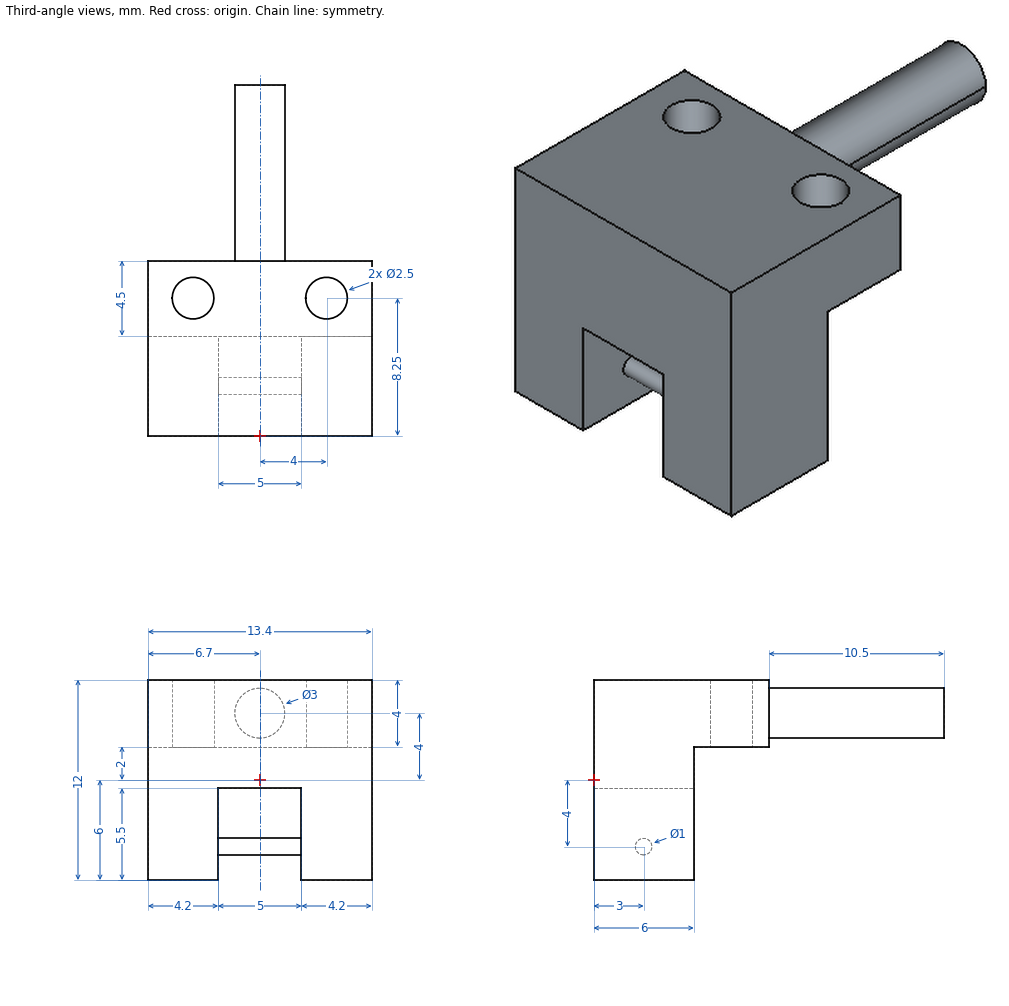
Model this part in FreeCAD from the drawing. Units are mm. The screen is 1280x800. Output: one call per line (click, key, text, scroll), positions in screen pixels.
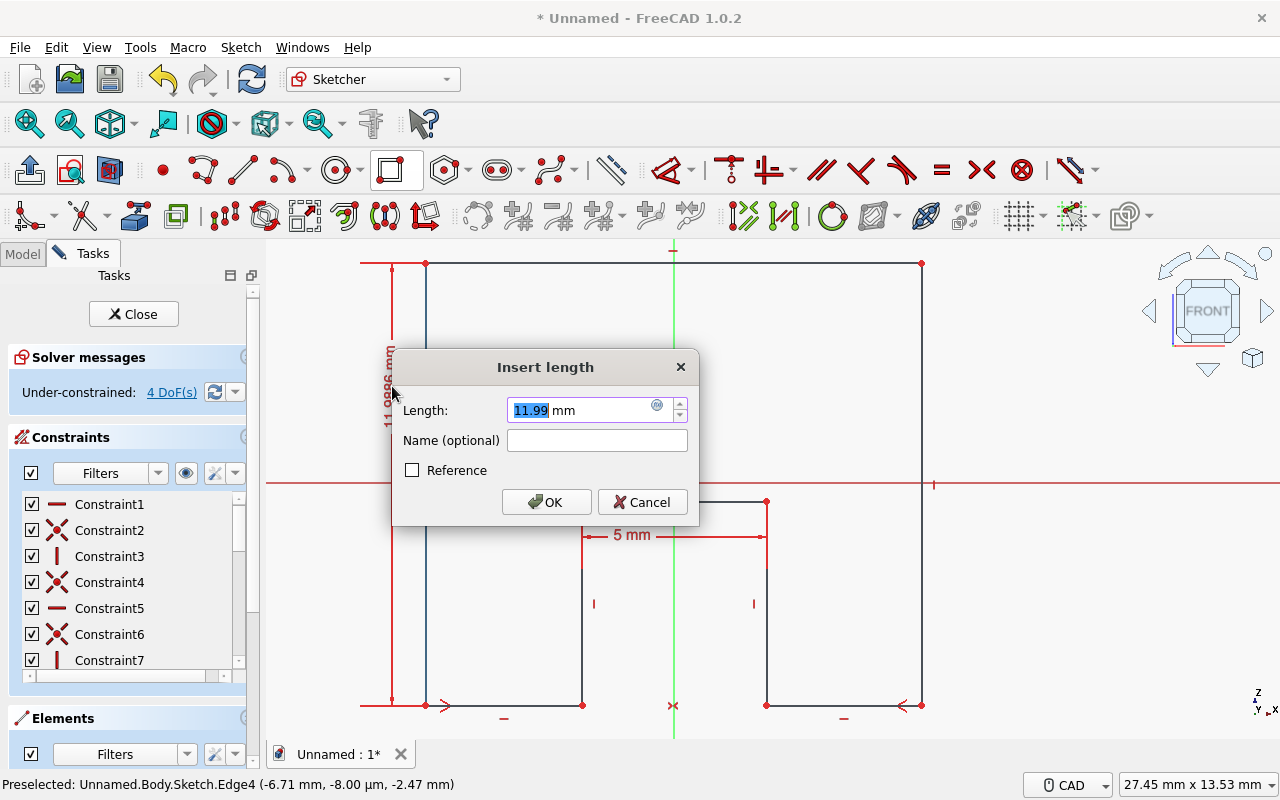
text(12)
key(Return)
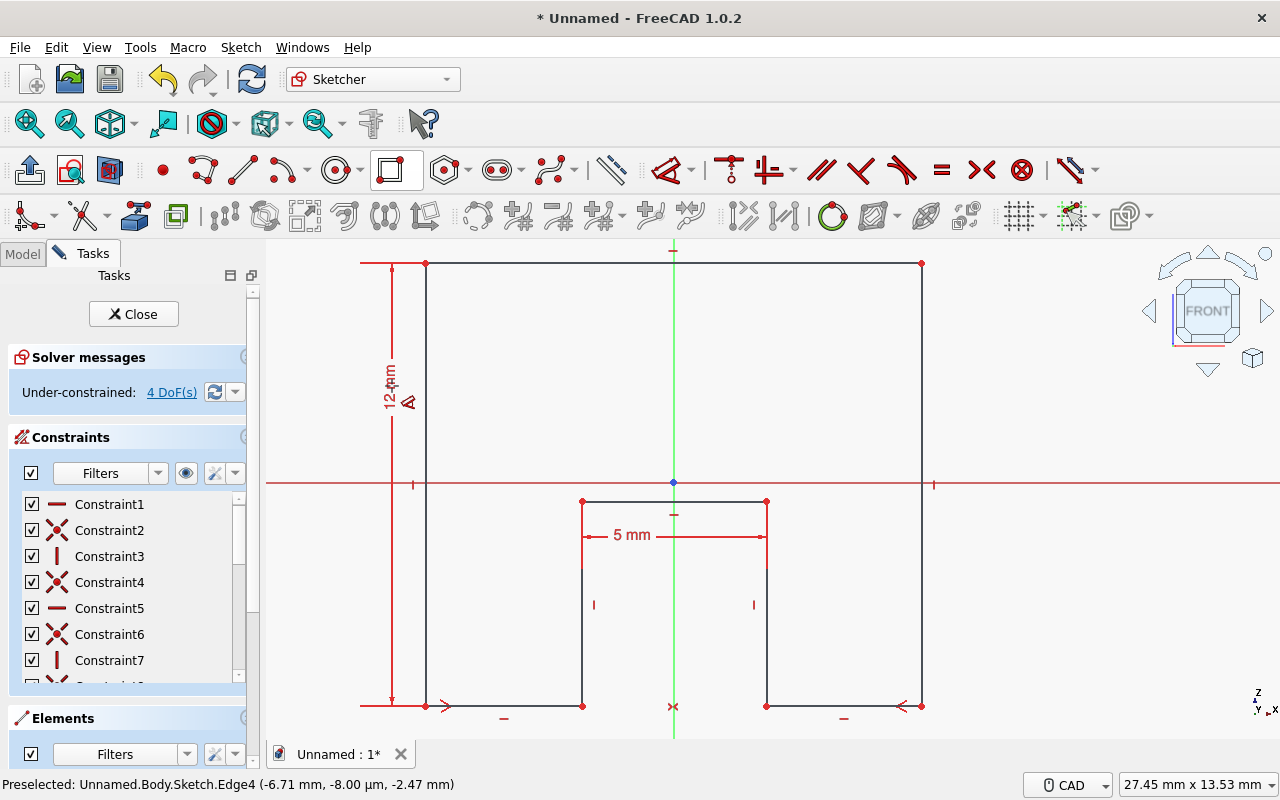
click(582, 706)
click(548, 595)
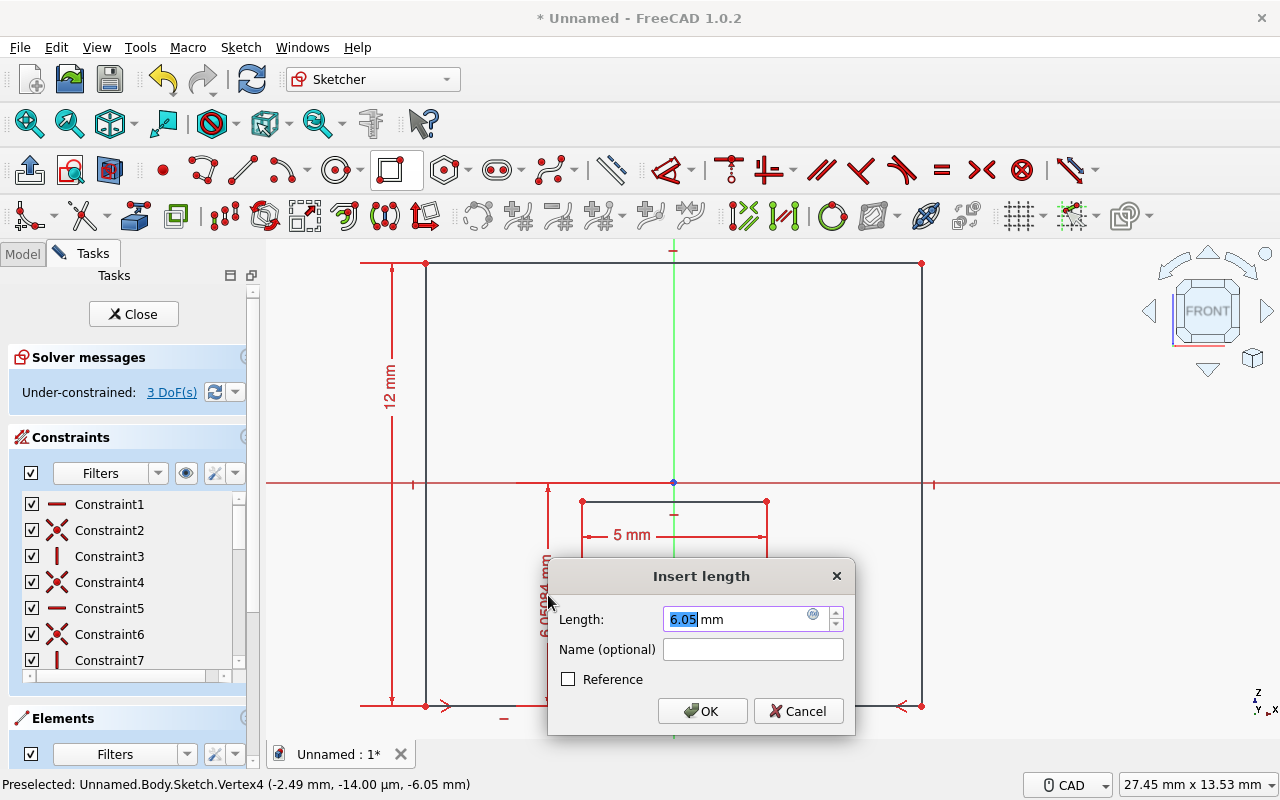
text(6)
key(Return)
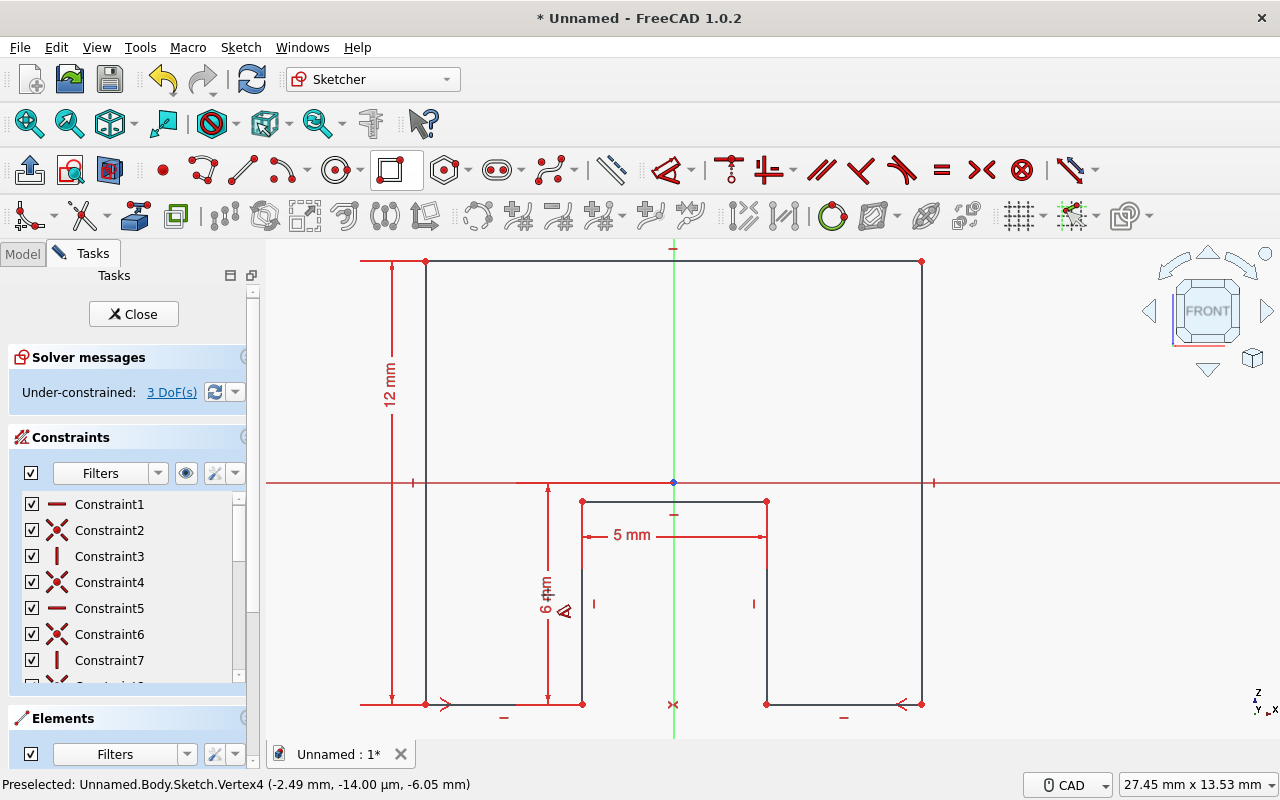
click(582, 563)
click(548, 557)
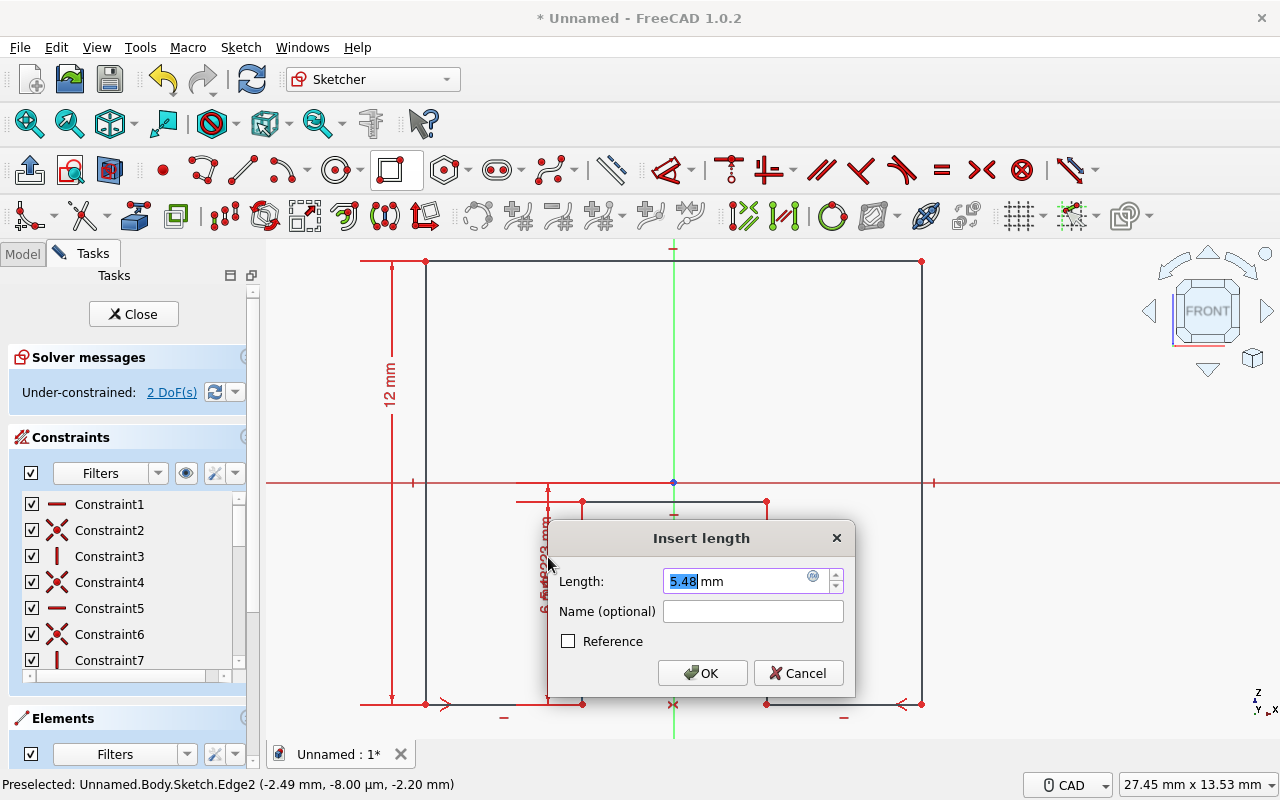
text(5.5)
key(Return)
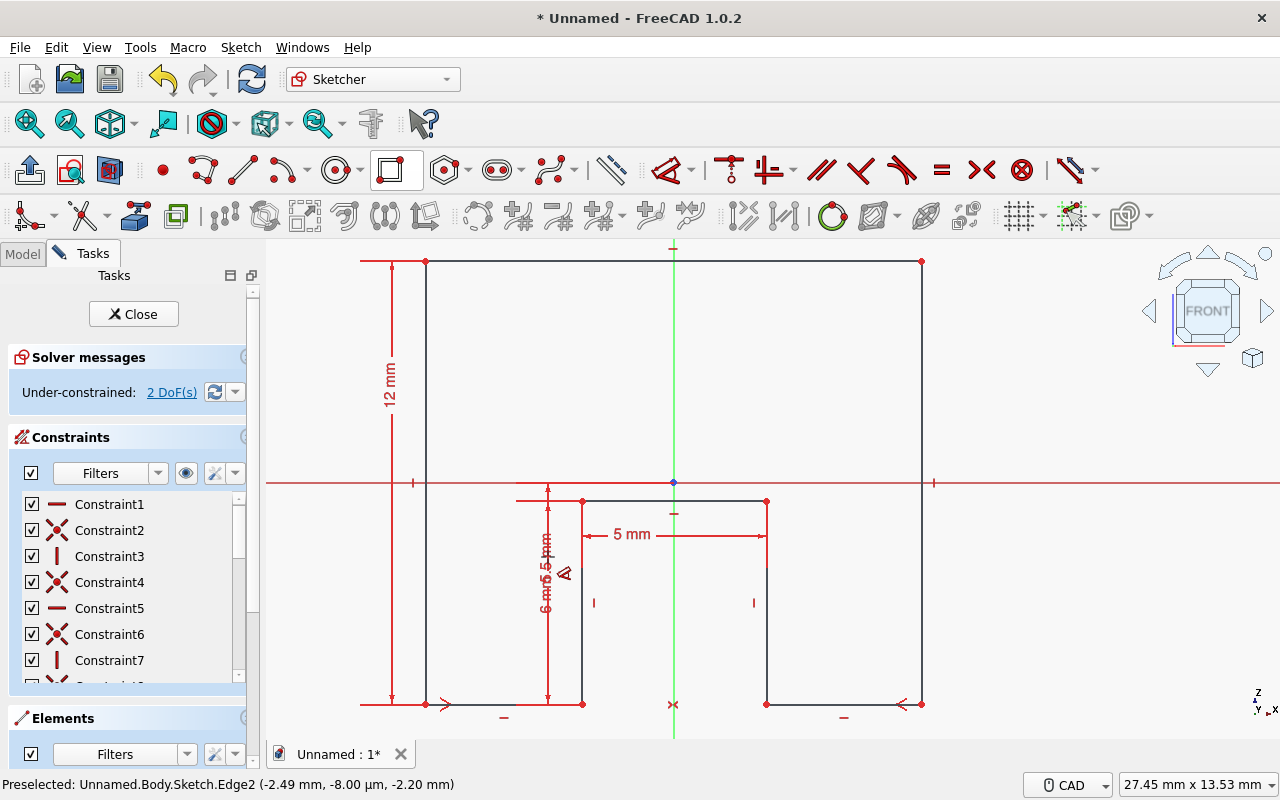
click(535, 705)
click(504, 671)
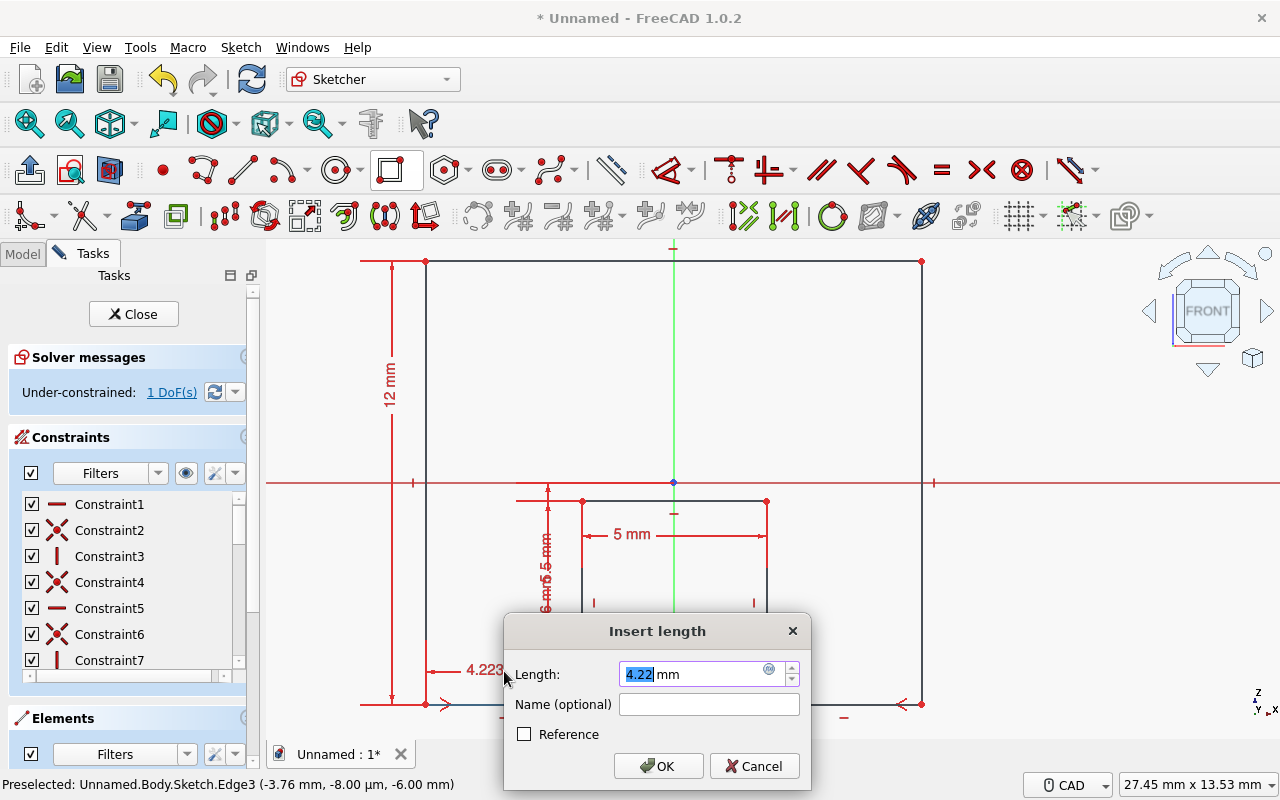
text(4.2)
key(Return)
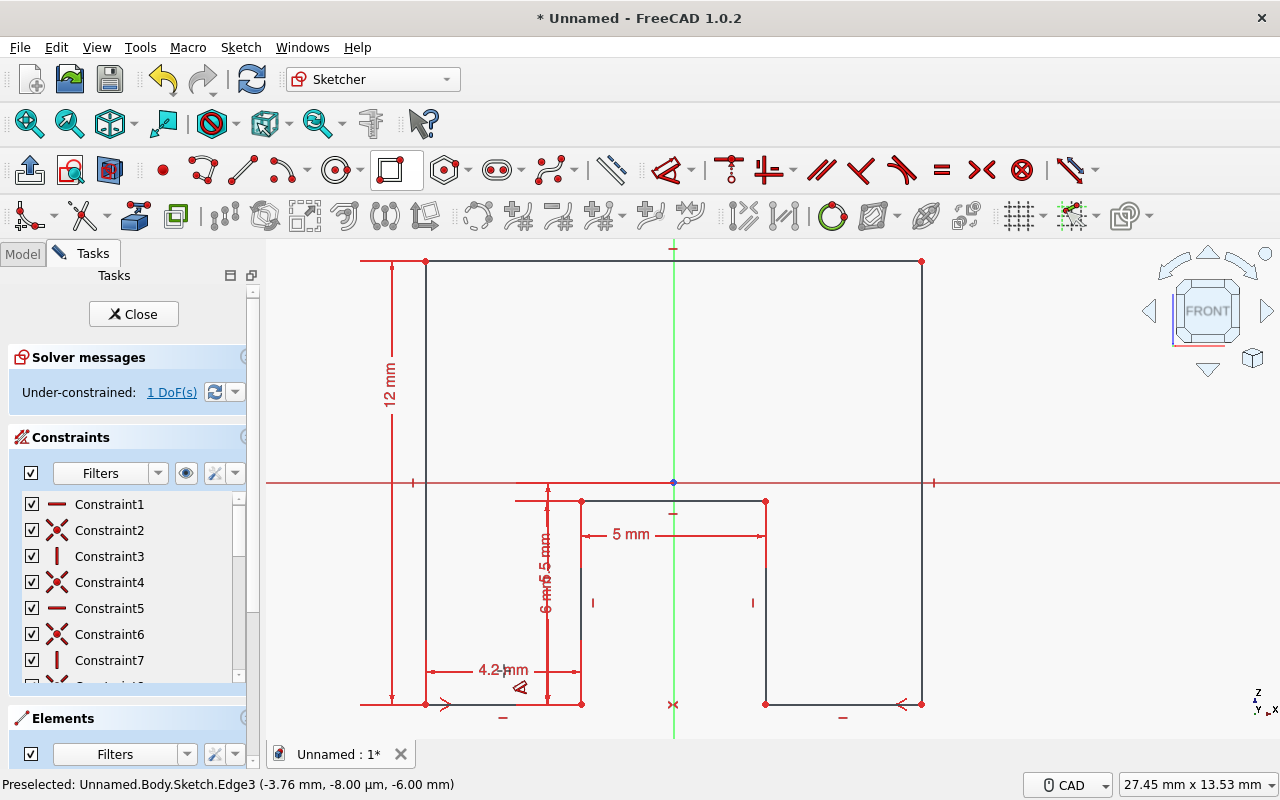
click(875, 705)
click(844, 671)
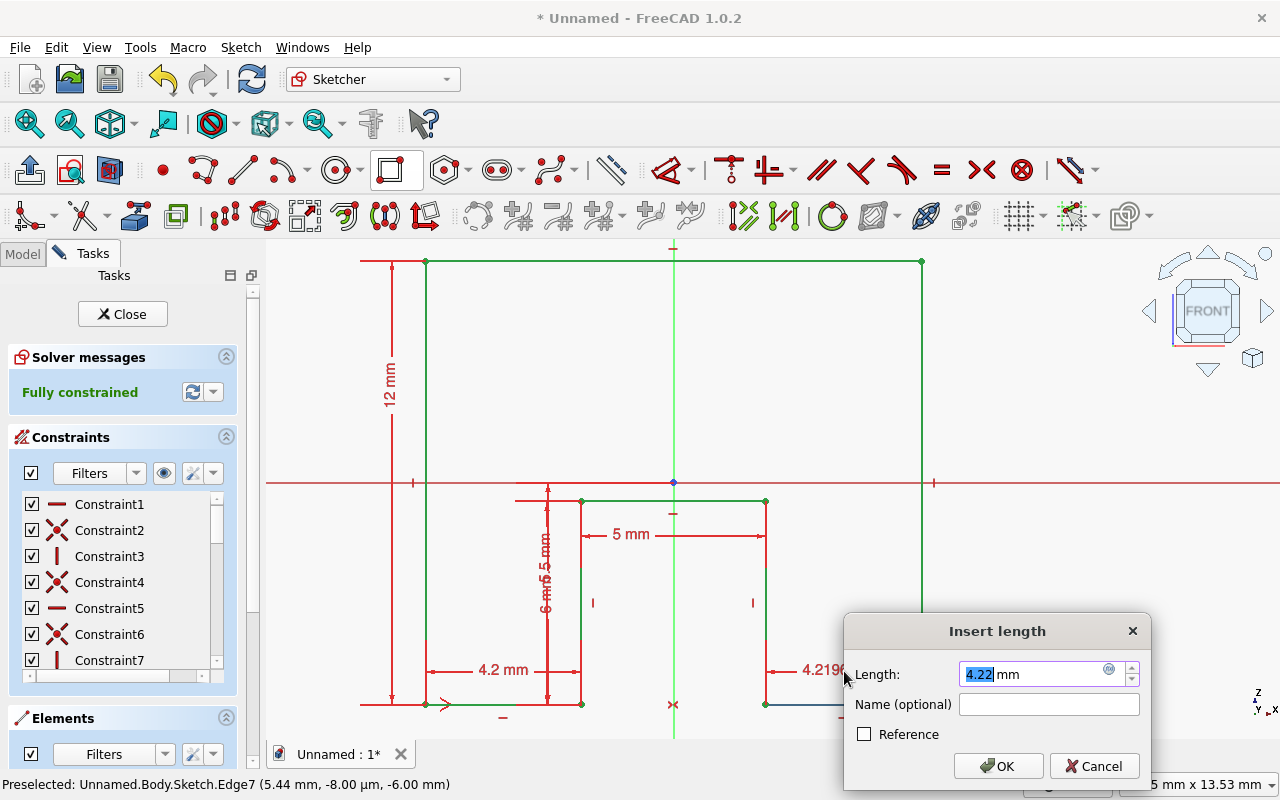
text(4.2)
key(Return)
key(Escape)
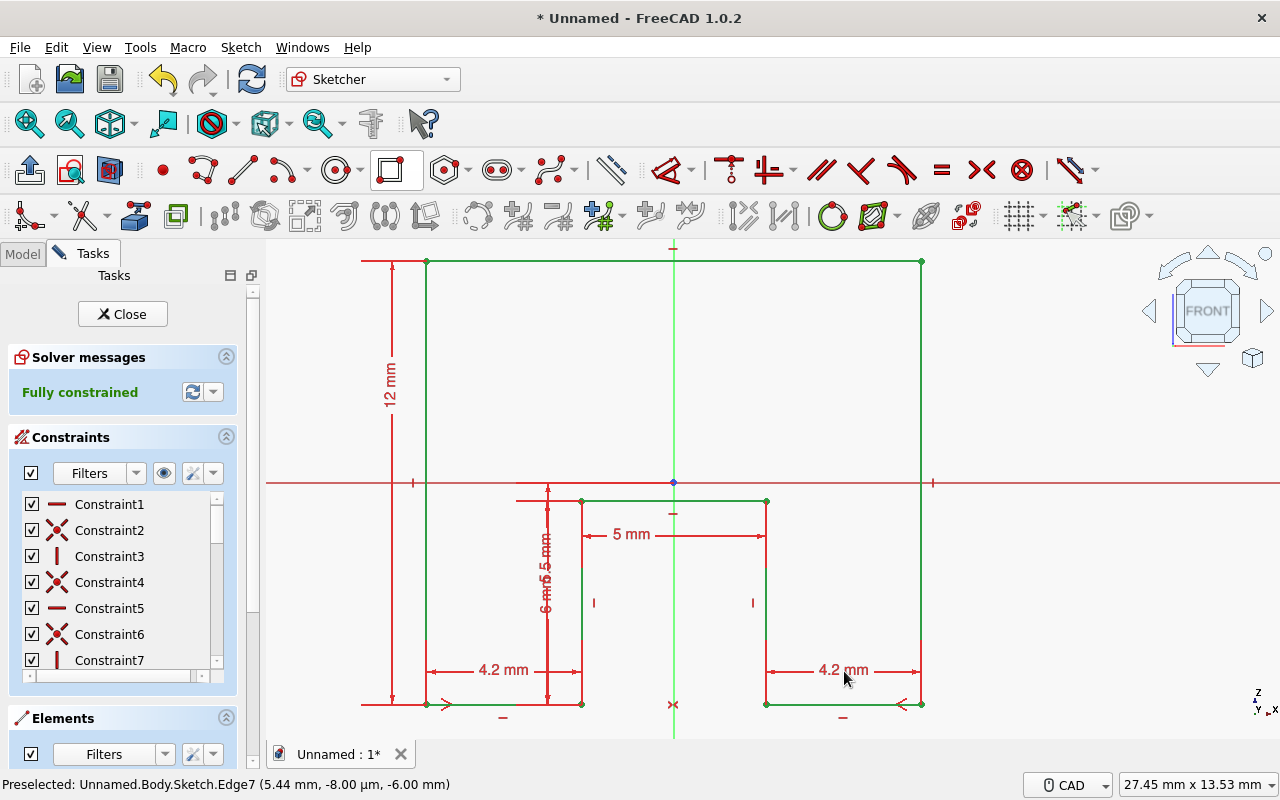
click(123, 314)